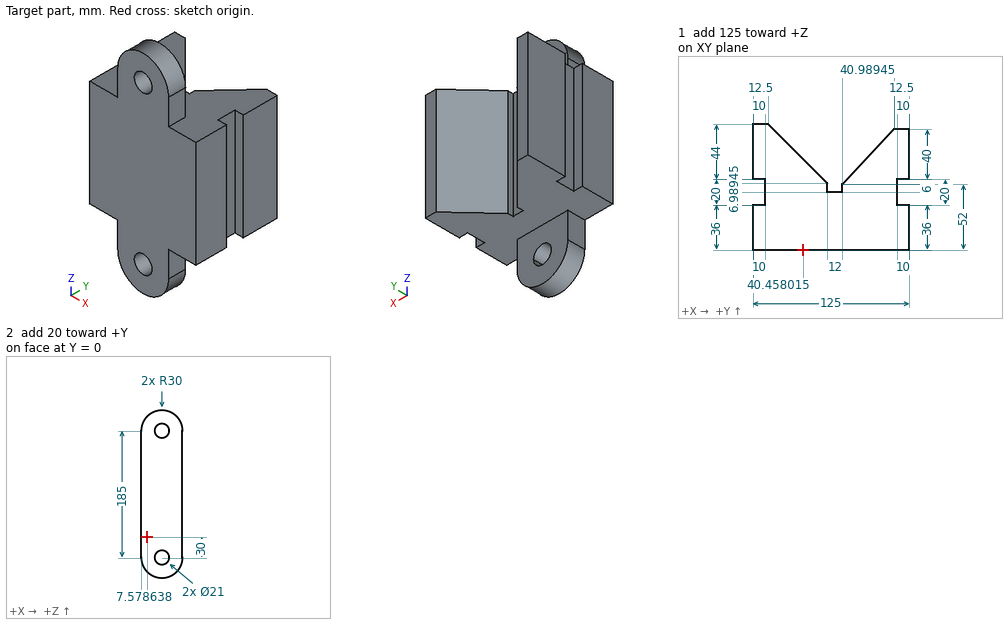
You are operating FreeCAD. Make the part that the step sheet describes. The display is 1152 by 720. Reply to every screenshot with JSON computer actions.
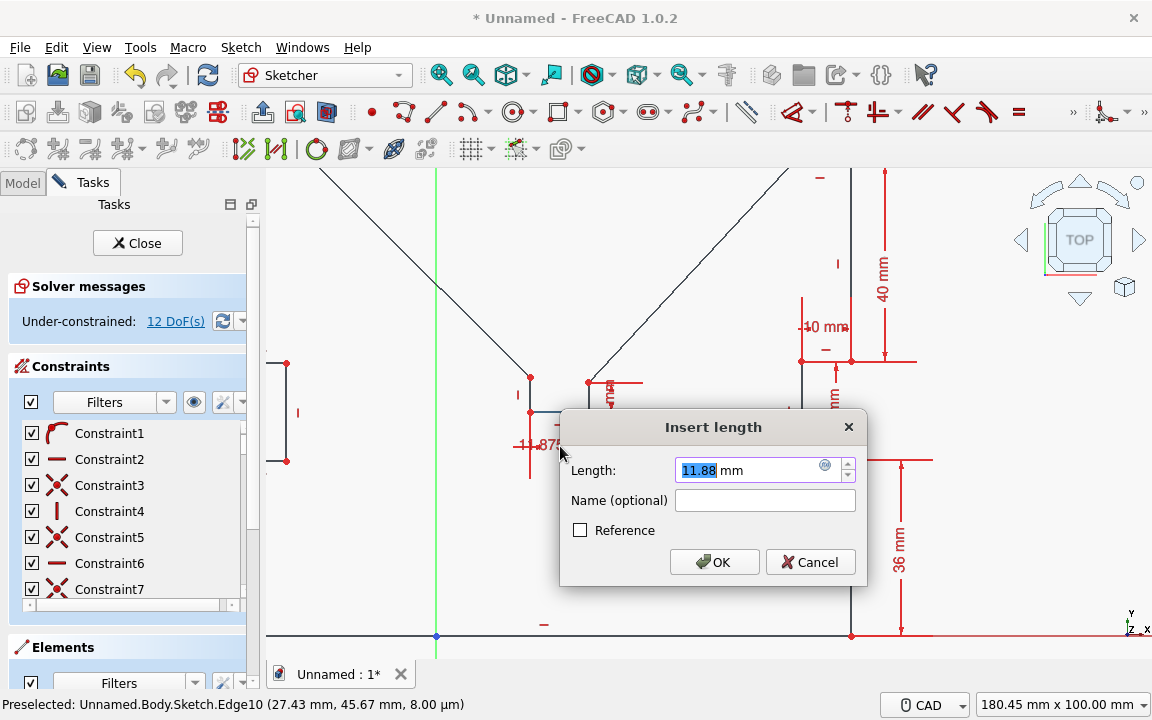
{"action": "type", "text": "12"}
{"action": "key", "text": "Return"}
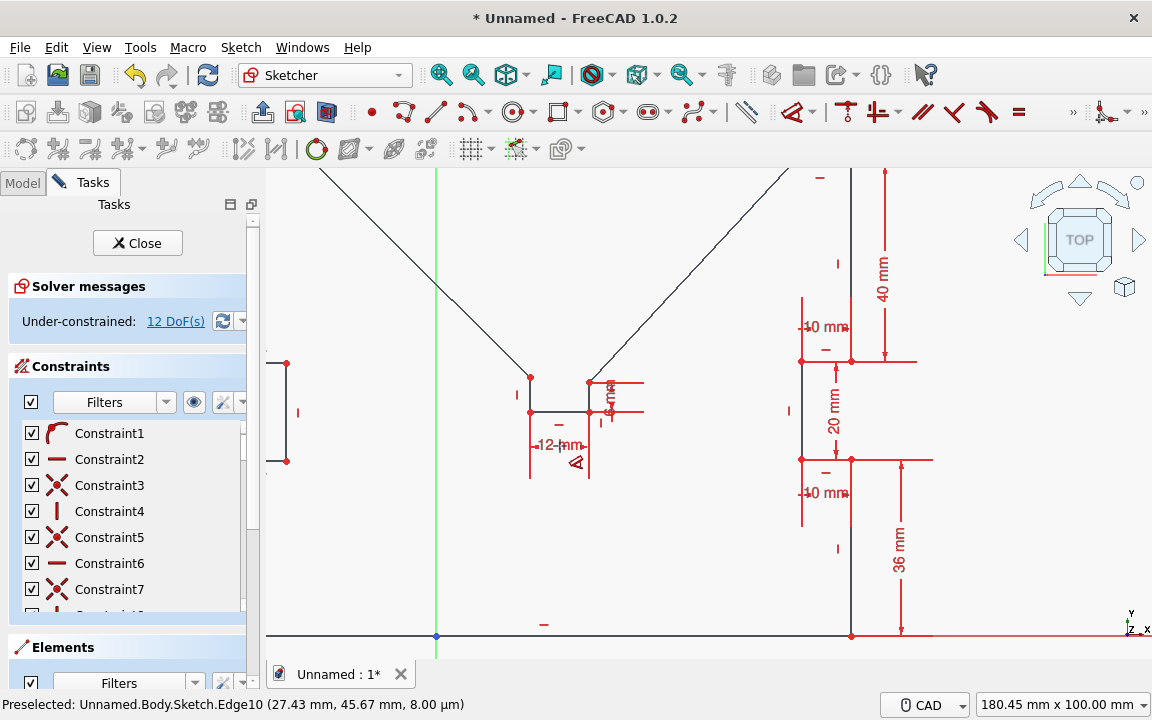
{"action": "scroll", "coordinate": [836, 459], "scroll_direction": "down", "scroll_amount": 2}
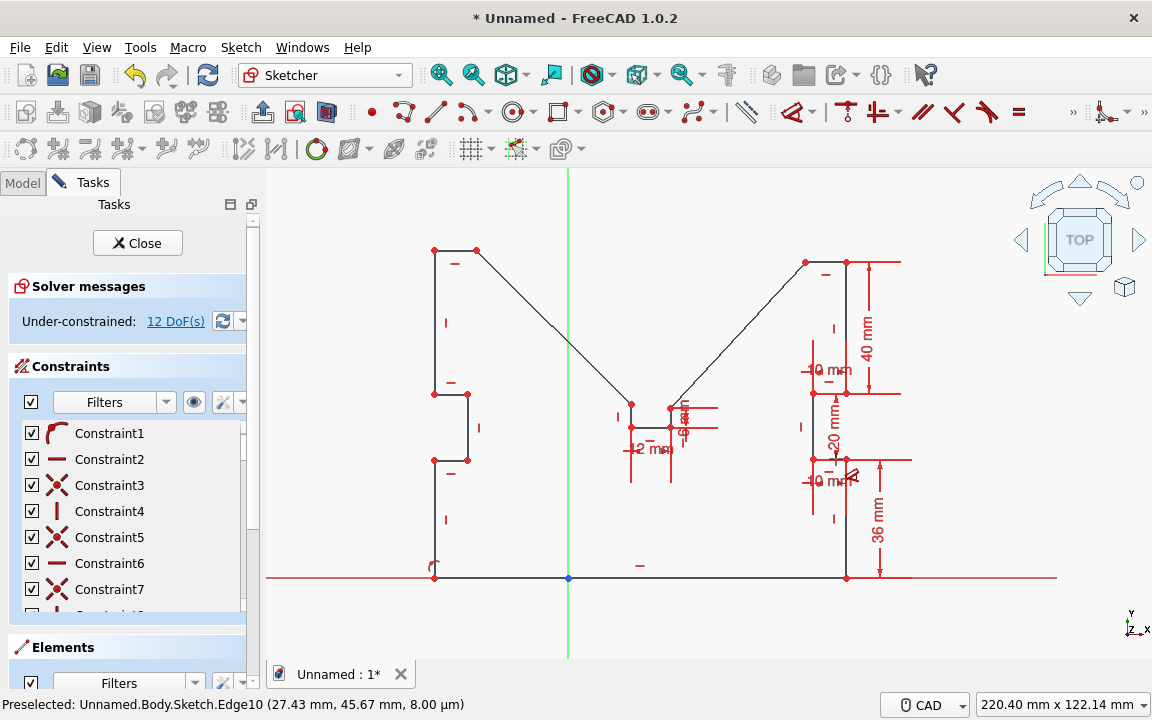
{"action": "left_click", "coordinate": [435, 294]}
{"action": "left_click", "coordinate": [401, 323]}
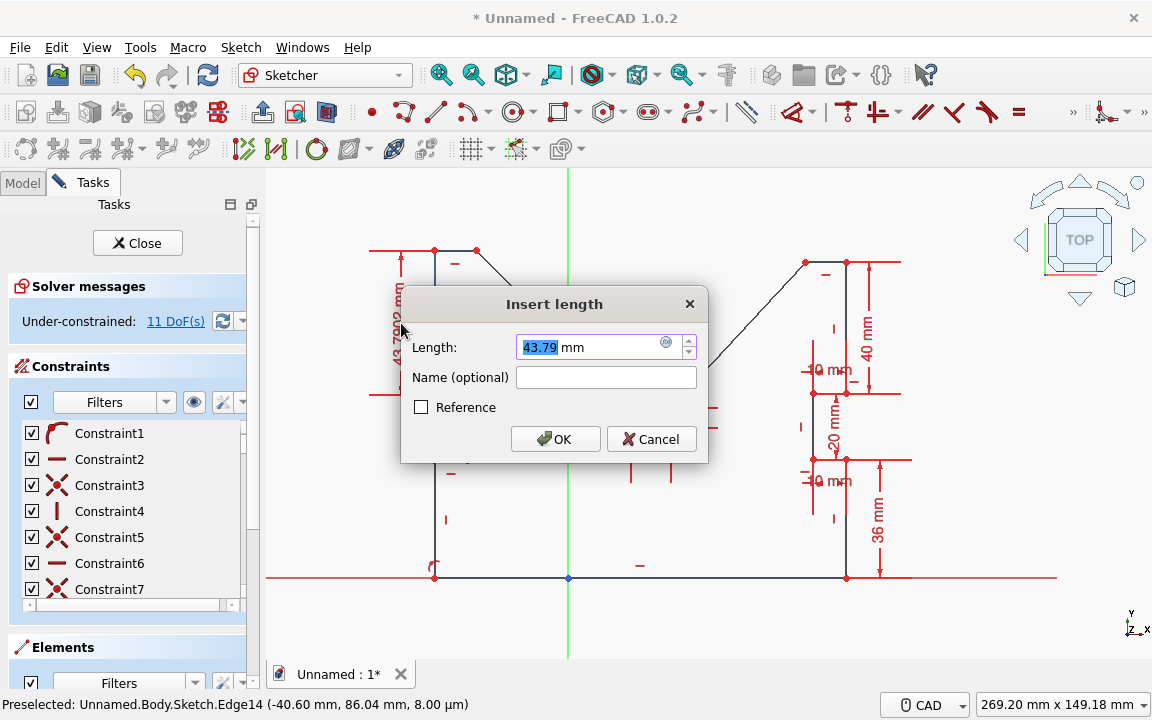
{"action": "type", "text": "44"}
{"action": "key", "text": "Return"}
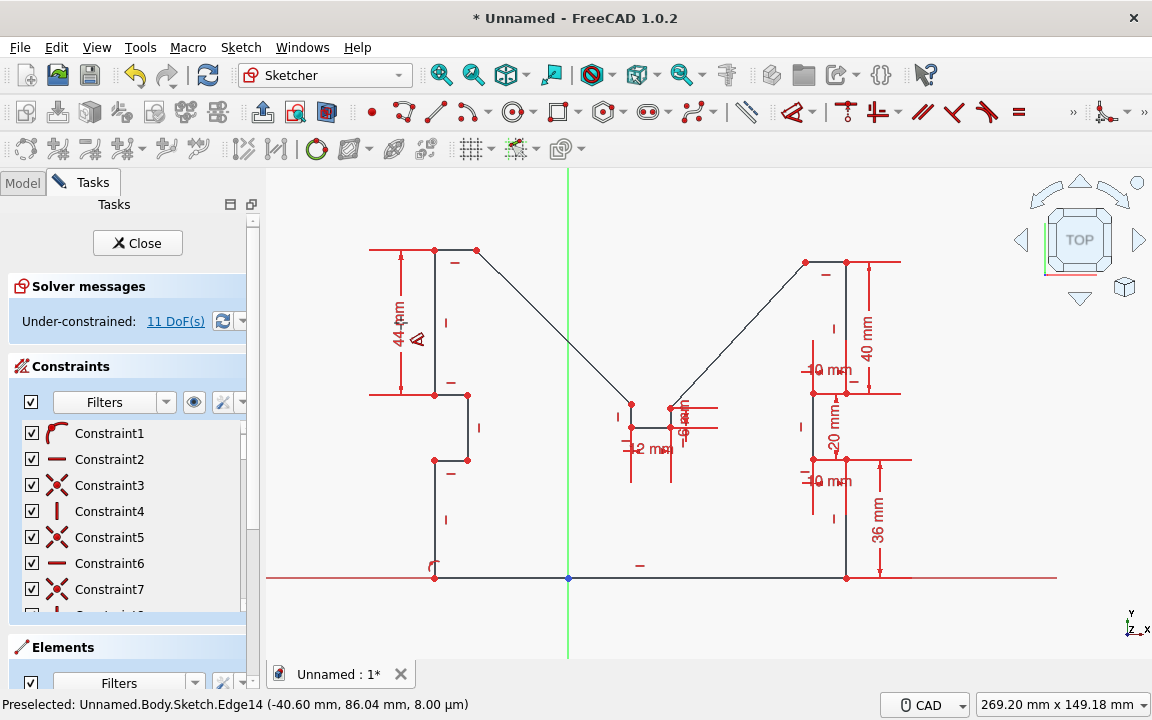
{"action": "scroll", "coordinate": [445, 395], "scroll_direction": "up", "scroll_amount": 2}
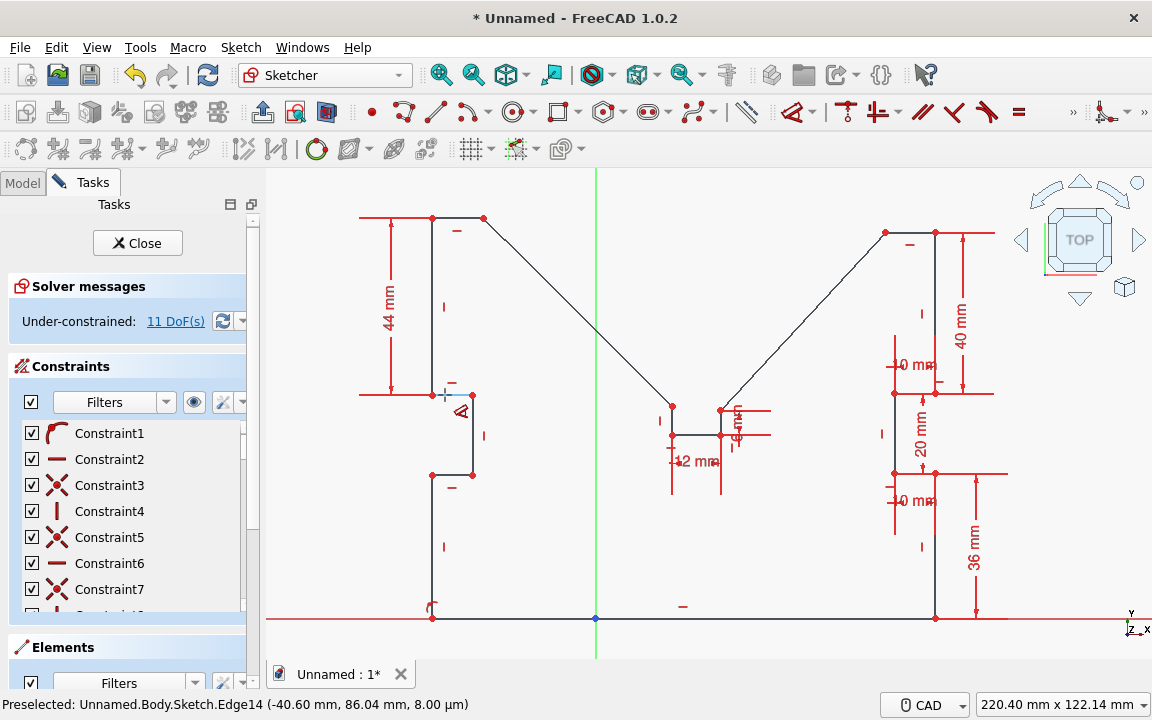
{"action": "left_click", "coordinate": [444, 395]}
{"action": "left_click", "coordinate": [454, 361]}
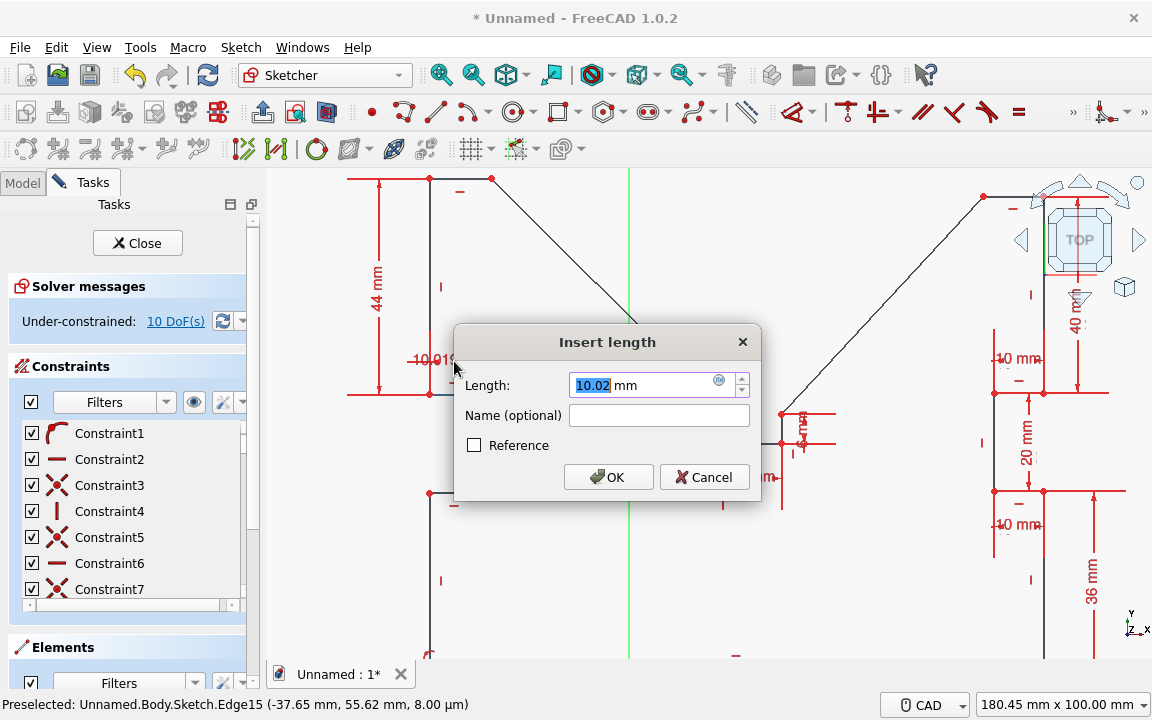
{"action": "type", "text": "10"}
{"action": "key", "text": "Return"}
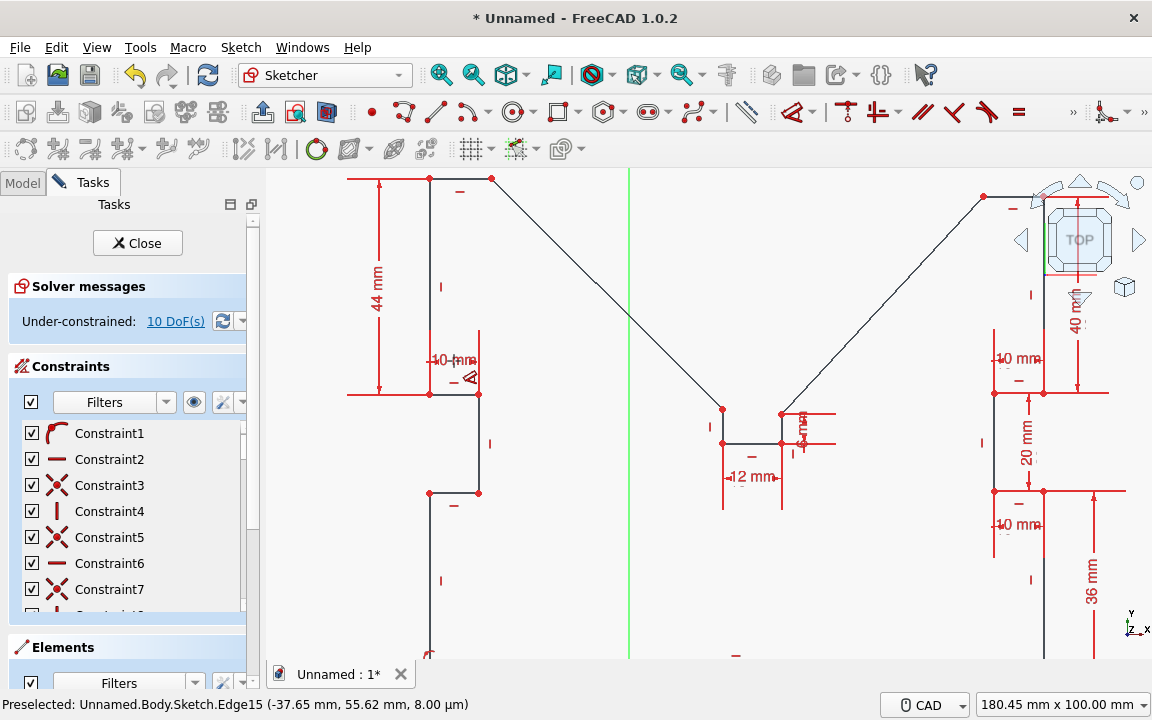
{"action": "left_click", "coordinate": [479, 424]}
{"action": "left_click", "coordinate": [445, 444]}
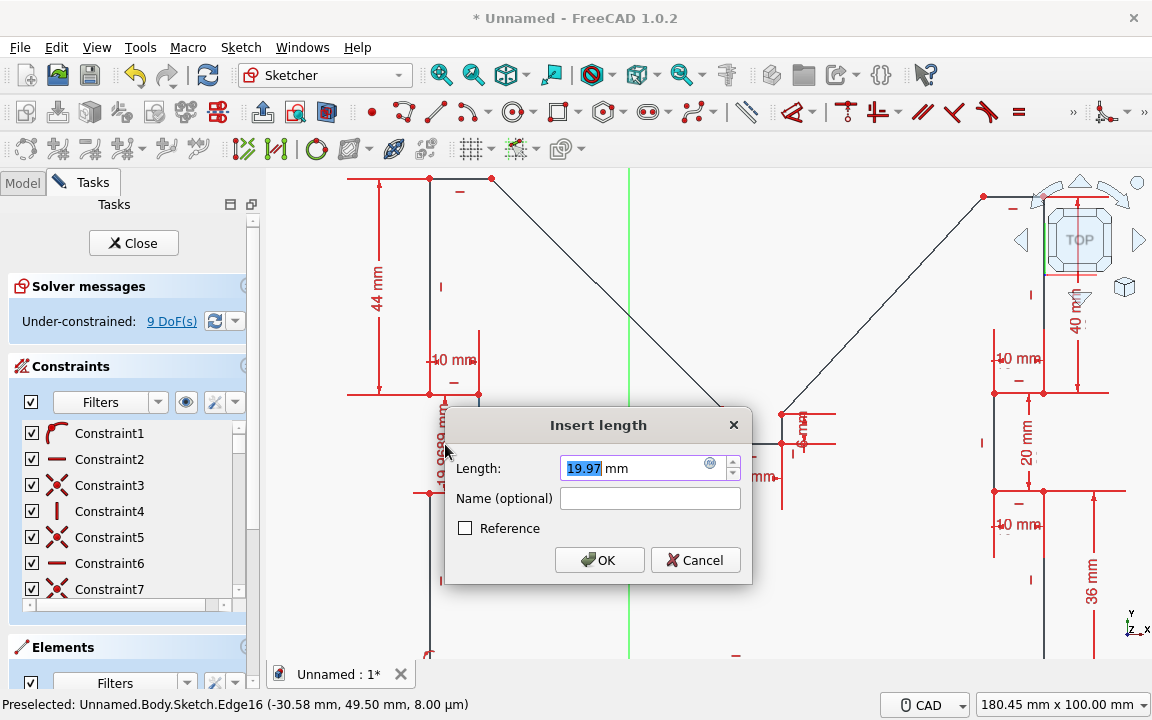
{"action": "type", "text": "20"}
{"action": "key", "text": "Return"}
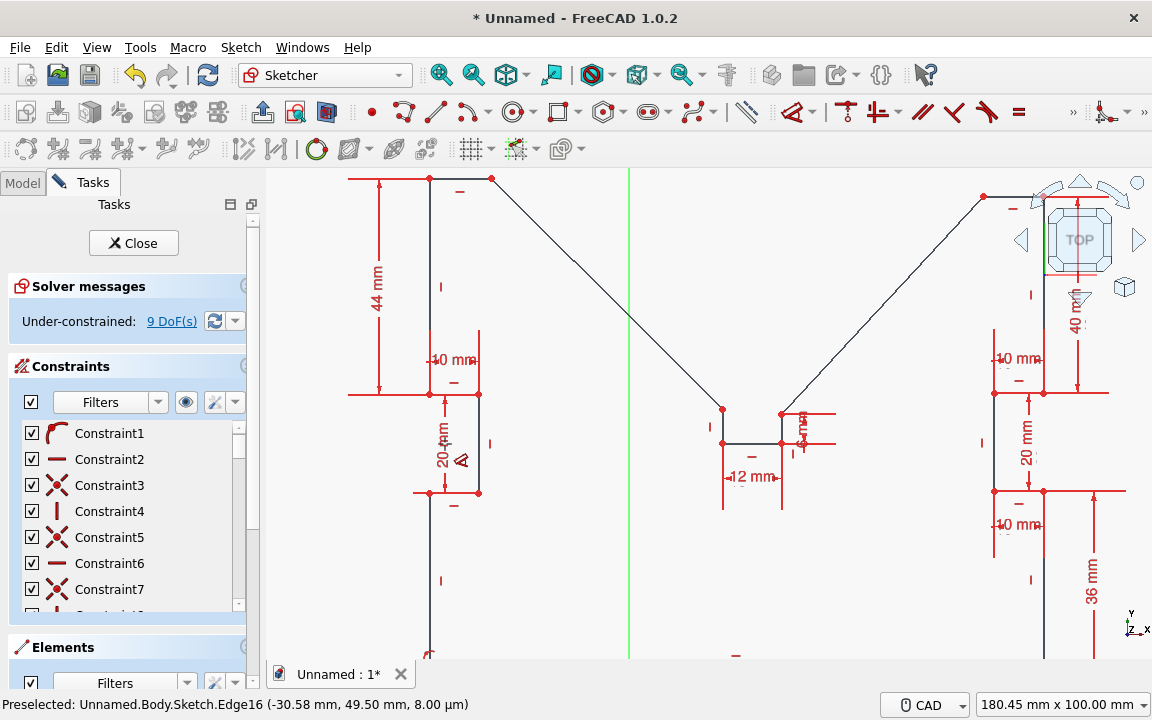
{"action": "left_click", "coordinate": [464, 493]}
{"action": "left_click", "coordinate": [454, 527]}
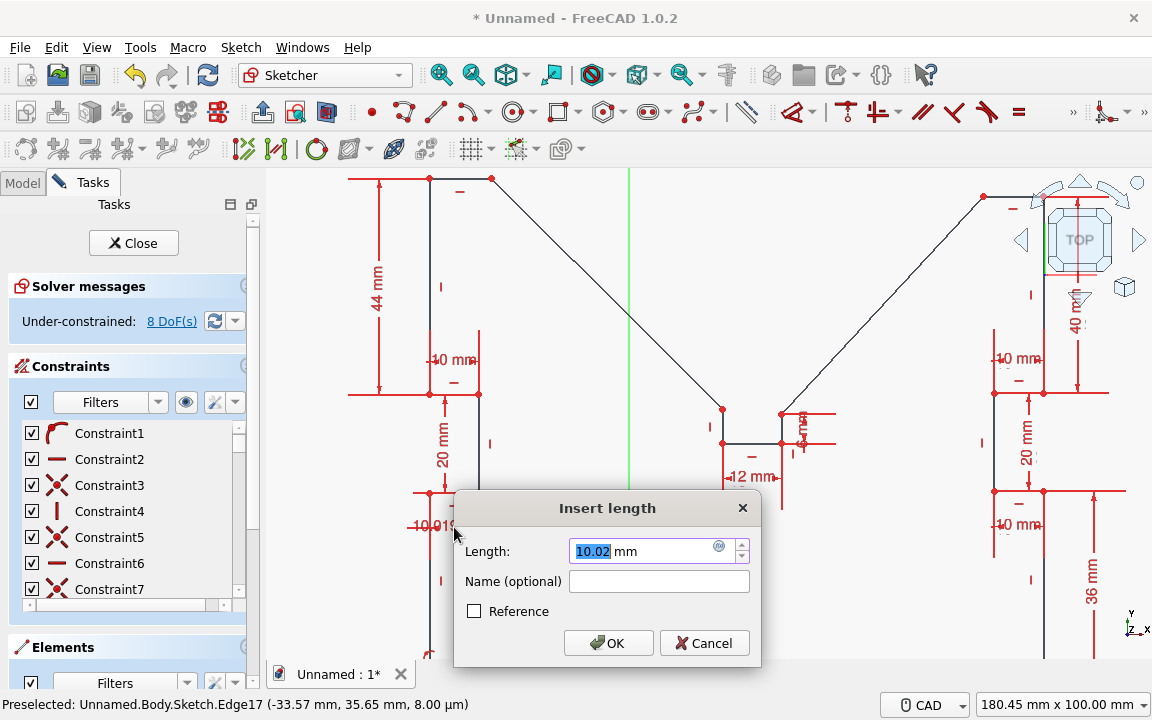
{"action": "type", "text": "10"}
{"action": "key", "text": "Return"}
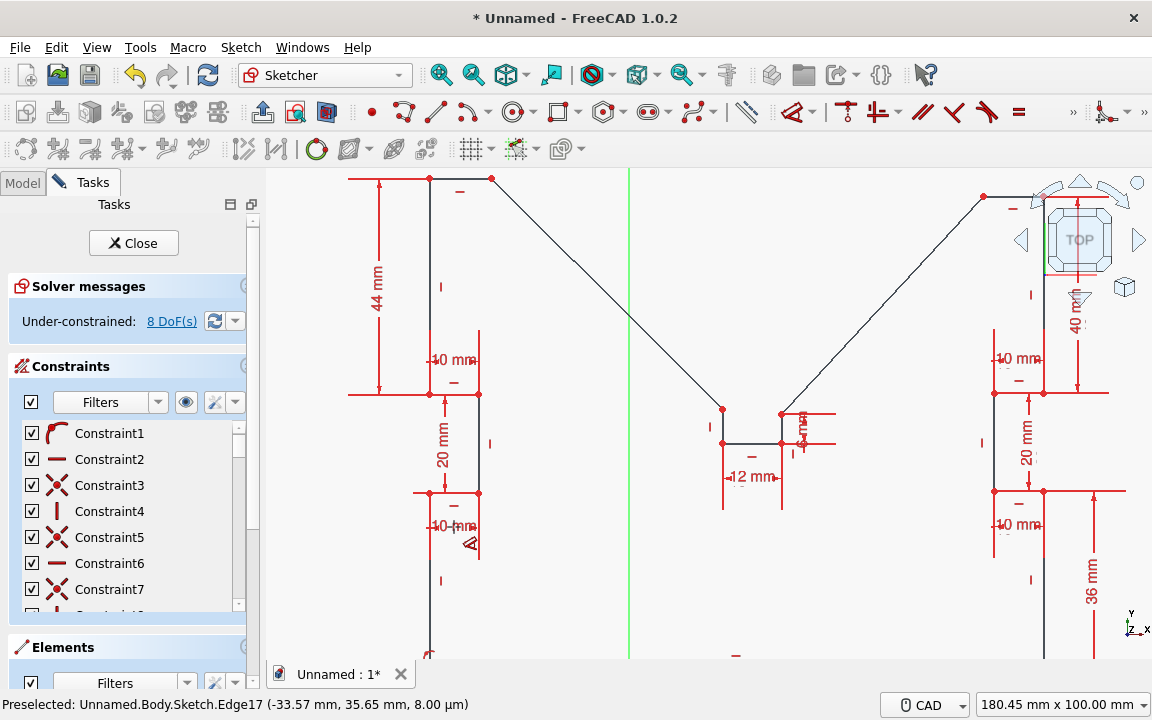
{"action": "left_click", "coordinate": [430, 546]}
{"action": "left_click", "coordinate": [396, 562]}